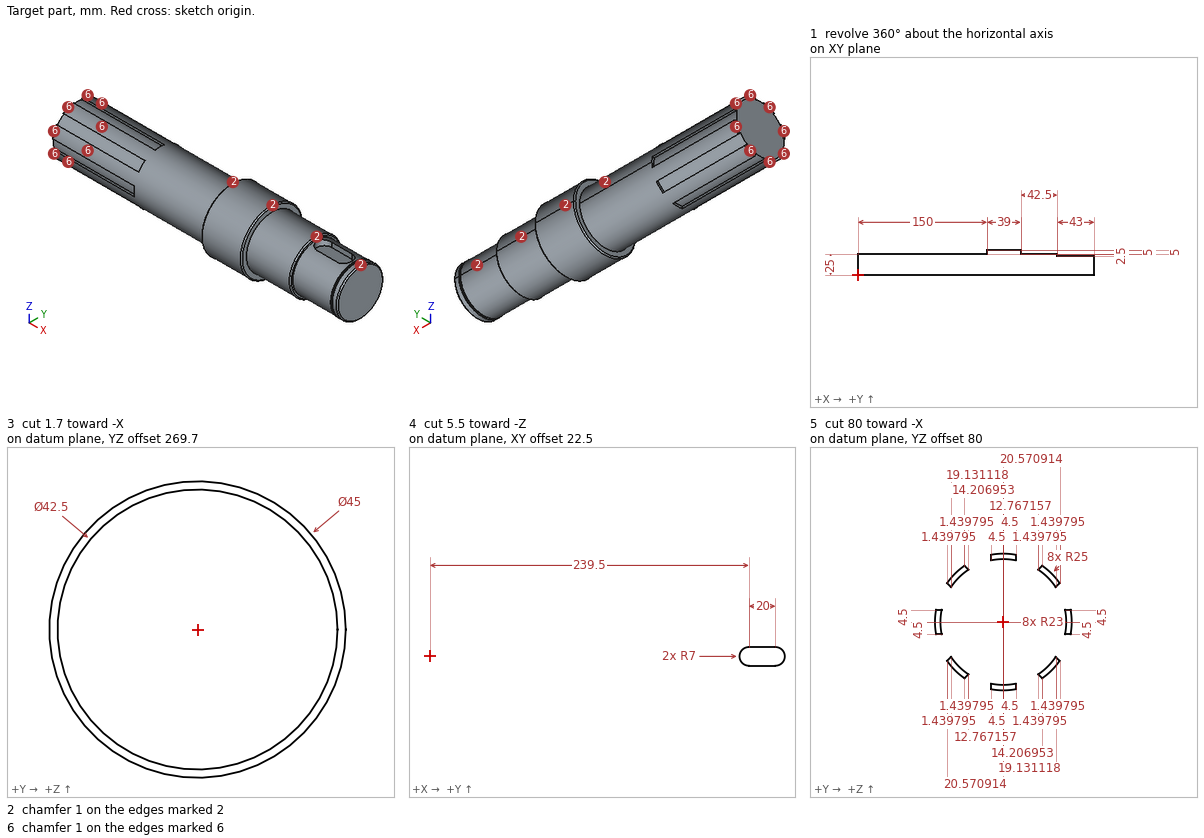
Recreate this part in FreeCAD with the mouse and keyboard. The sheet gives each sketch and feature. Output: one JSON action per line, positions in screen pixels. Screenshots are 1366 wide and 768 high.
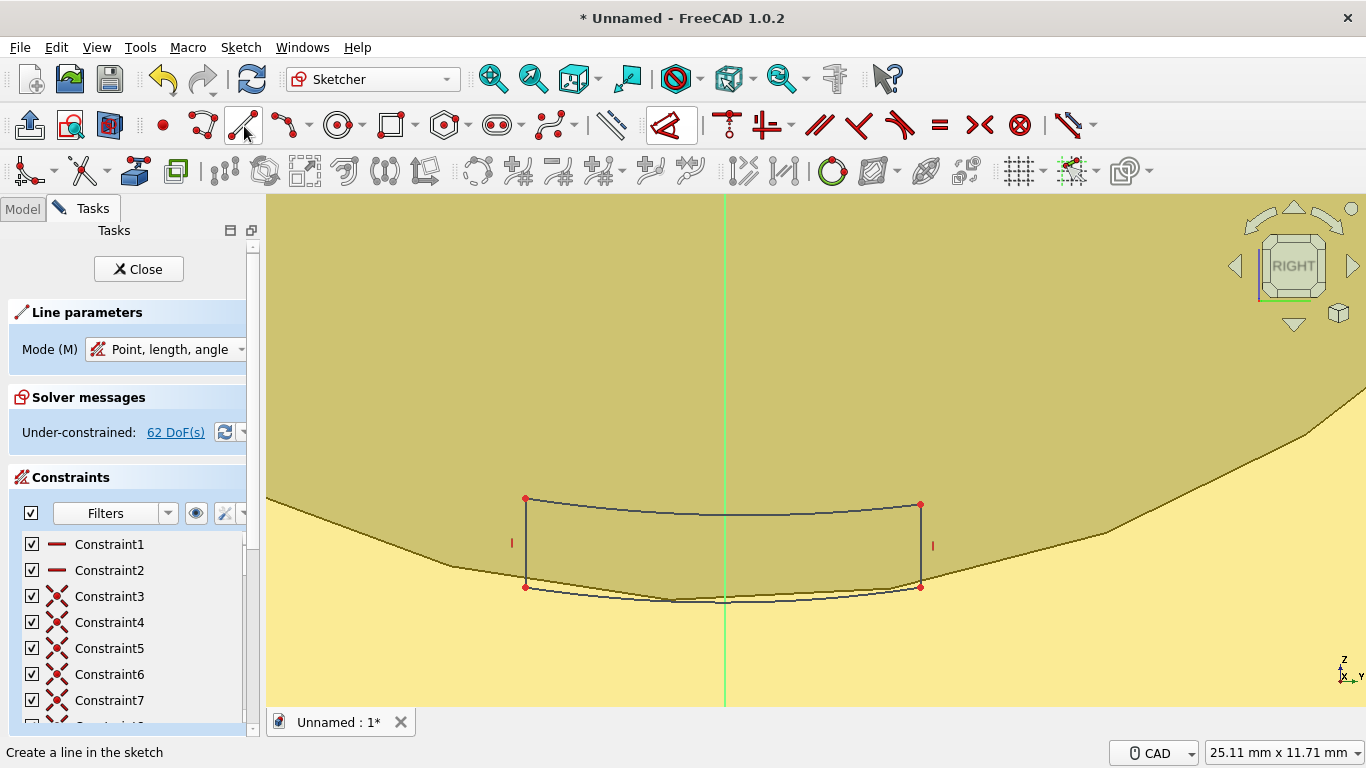
{"action": "scroll", "coordinate": [751, 598], "scroll_direction": "down", "scroll_amount": 10}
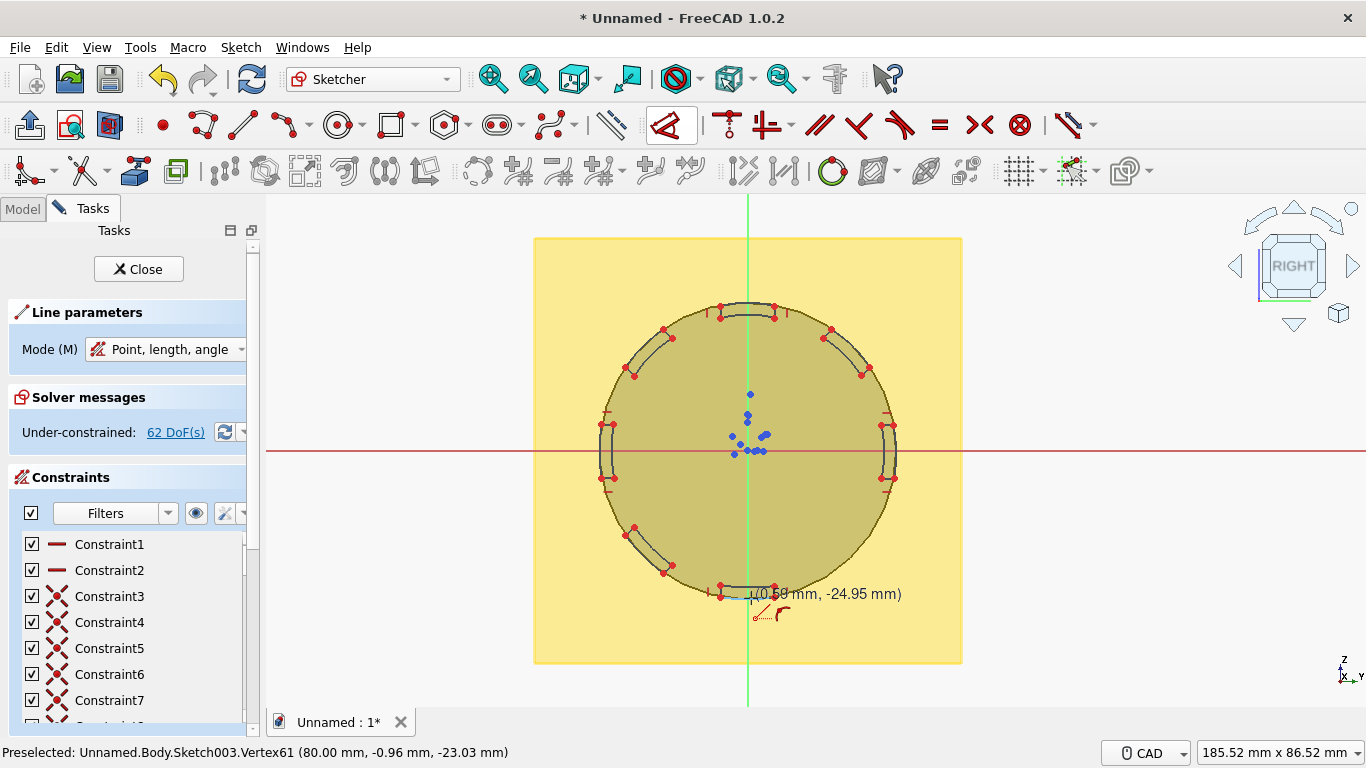
{"action": "left_click", "coordinate": [861, 527]}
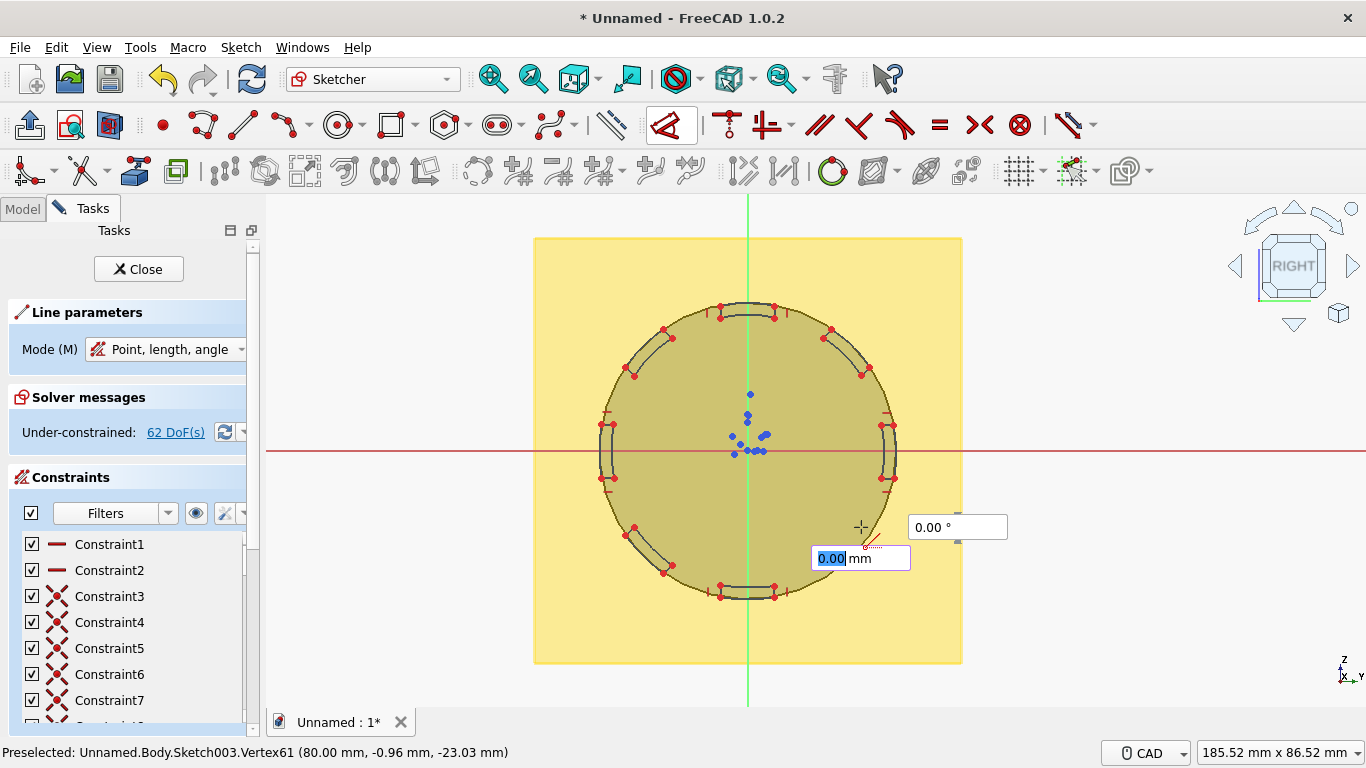
{"action": "scroll", "coordinate": [870, 535], "scroll_direction": "up", "scroll_amount": 2}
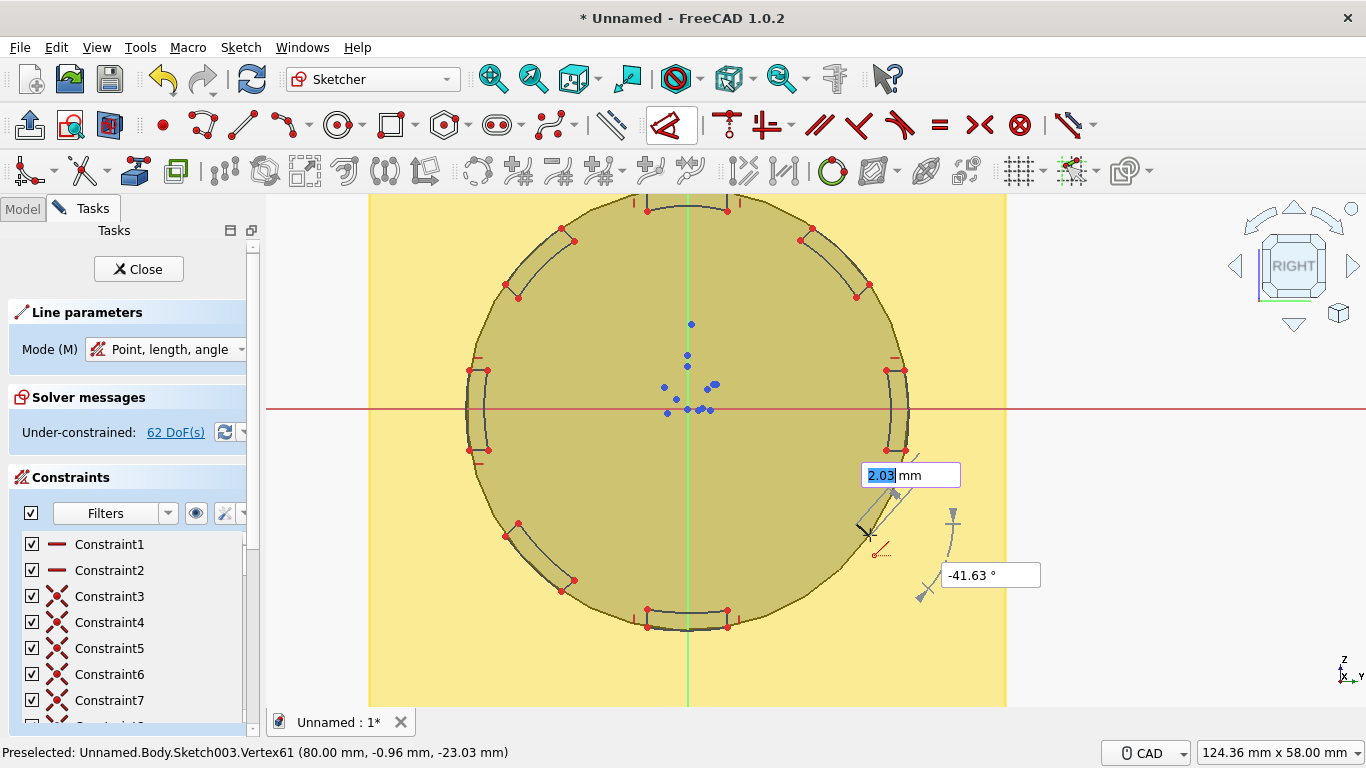
{"action": "left_click", "coordinate": [870, 535]}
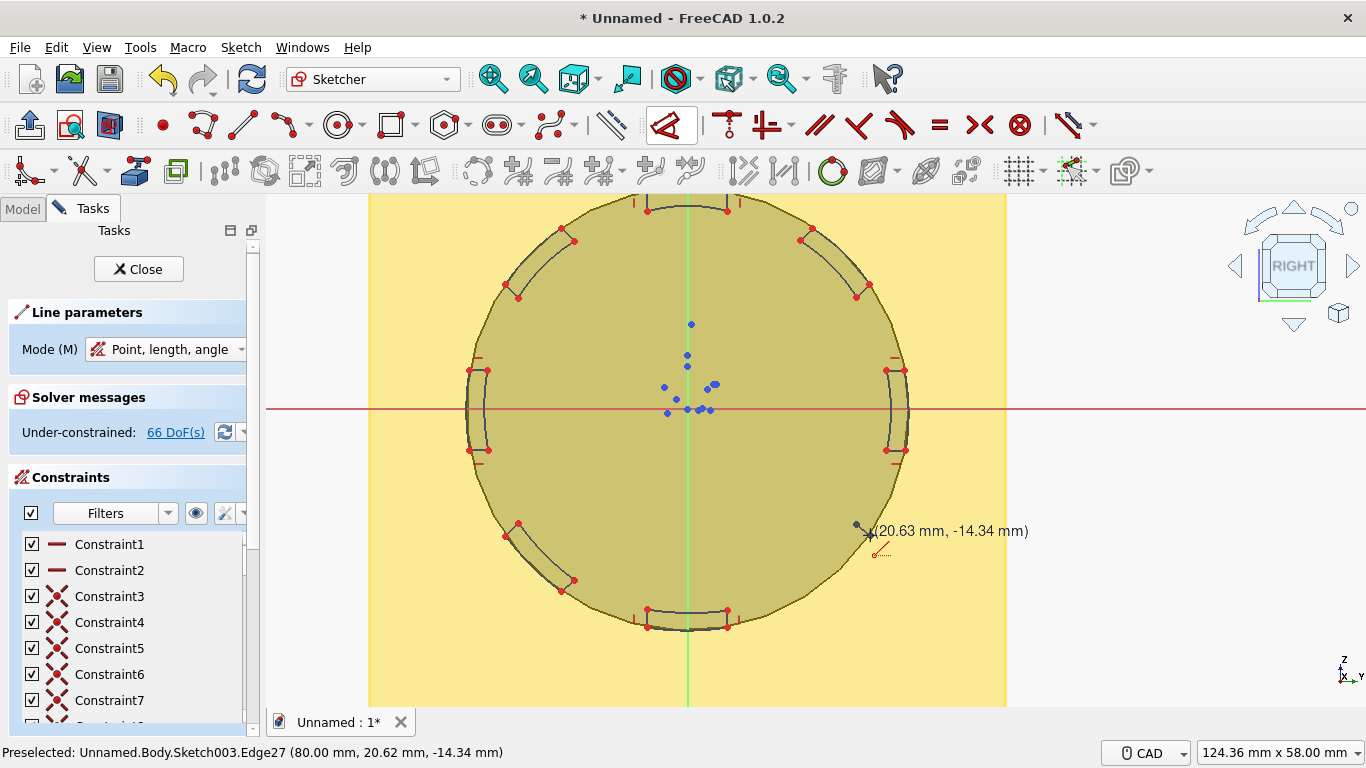
{"action": "left_click", "coordinate": [813, 591]}
{"action": "left_click", "coordinate": [800, 578]}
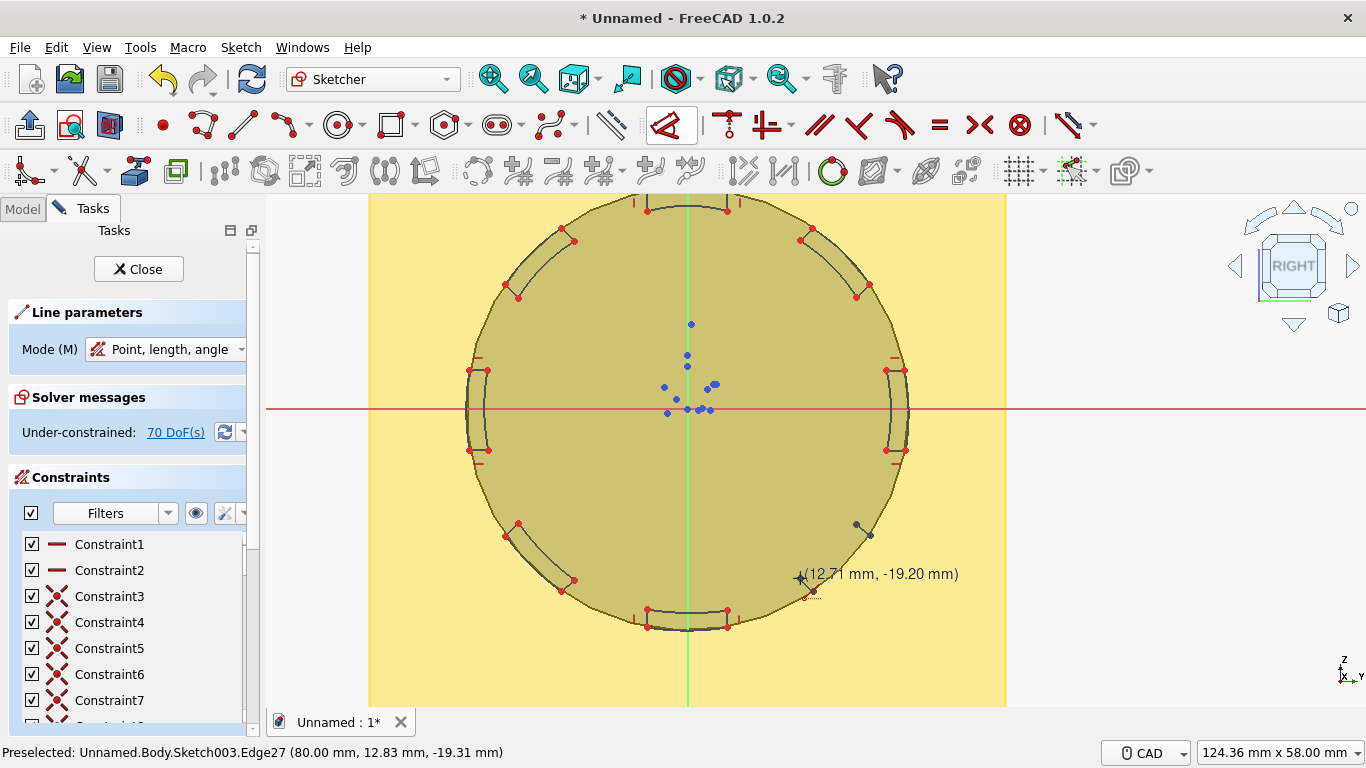
{"action": "left_click", "coordinate": [284, 126]}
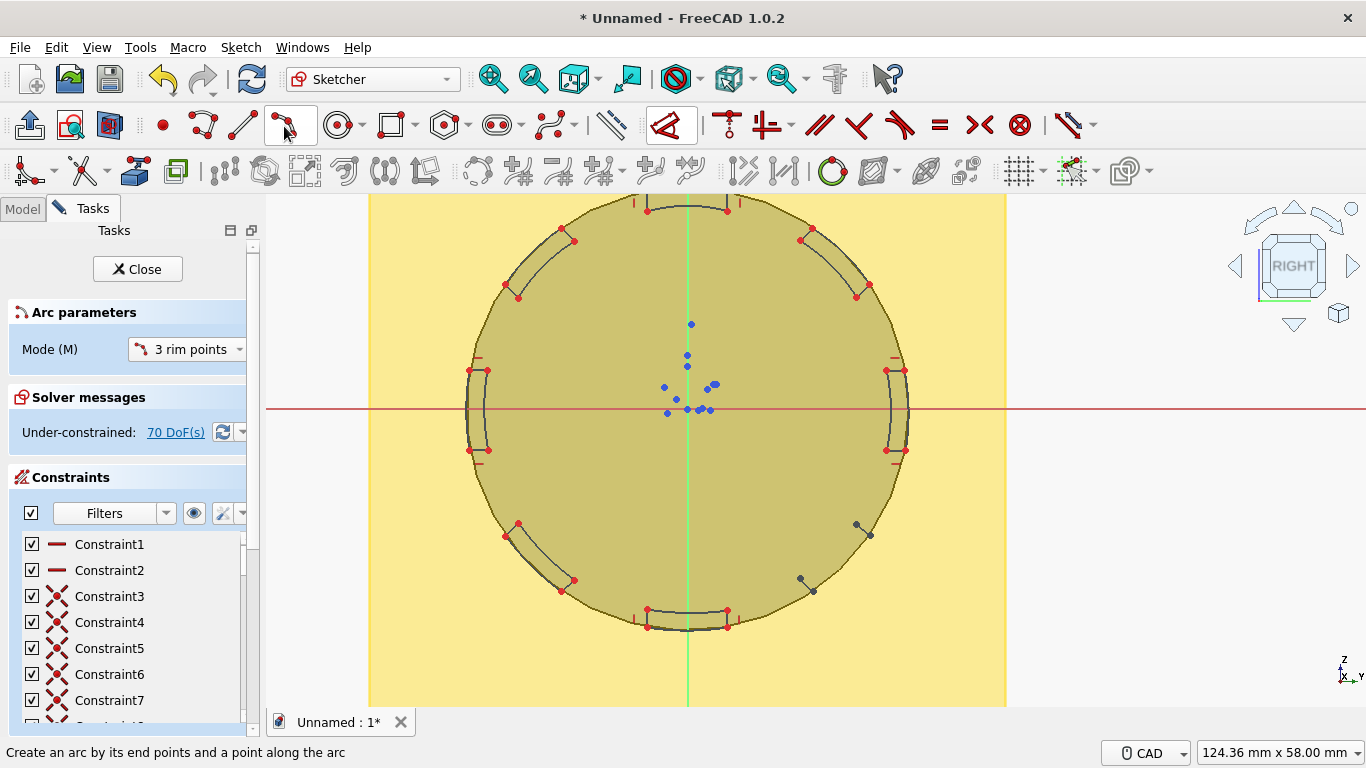
{"action": "scroll", "coordinate": [870, 535], "scroll_direction": "up", "scroll_amount": 3}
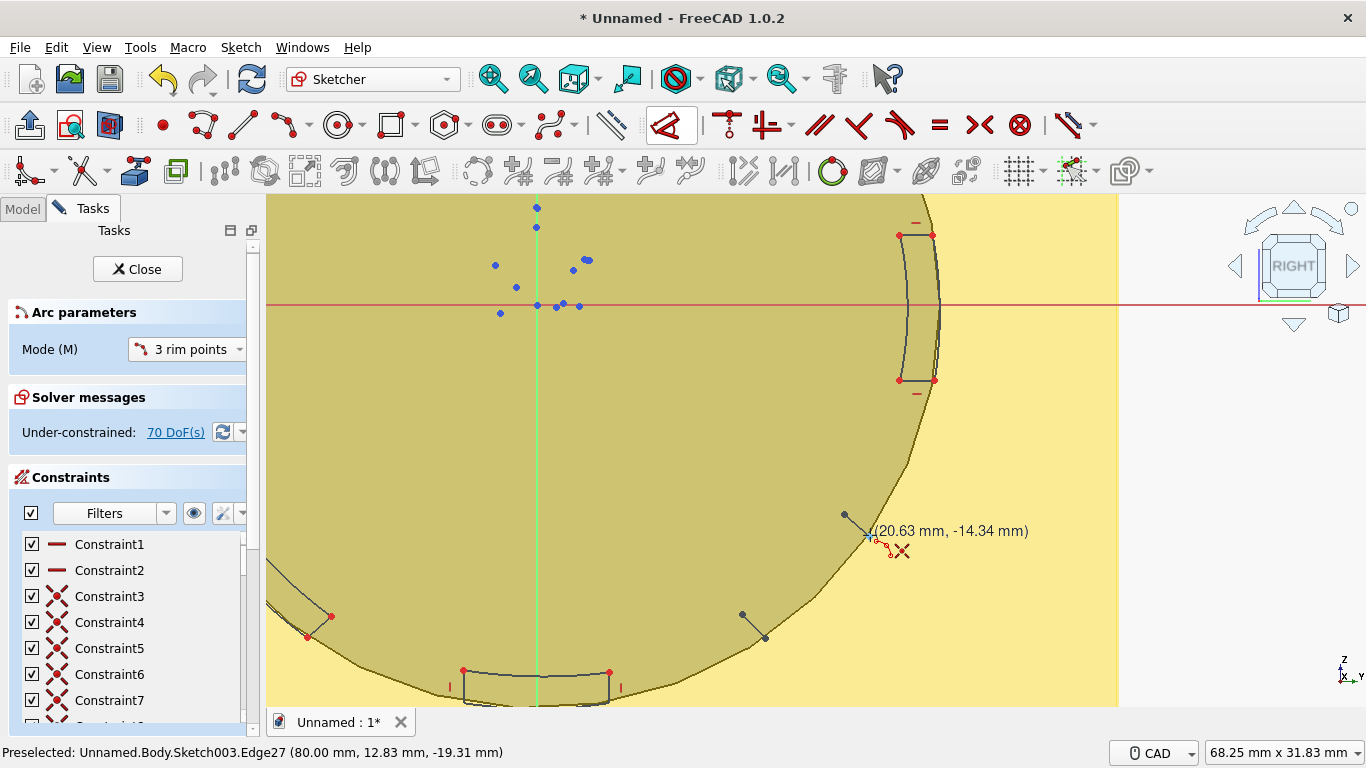
{"action": "left_click", "coordinate": [870, 536]}
{"action": "left_click", "coordinate": [766, 638]}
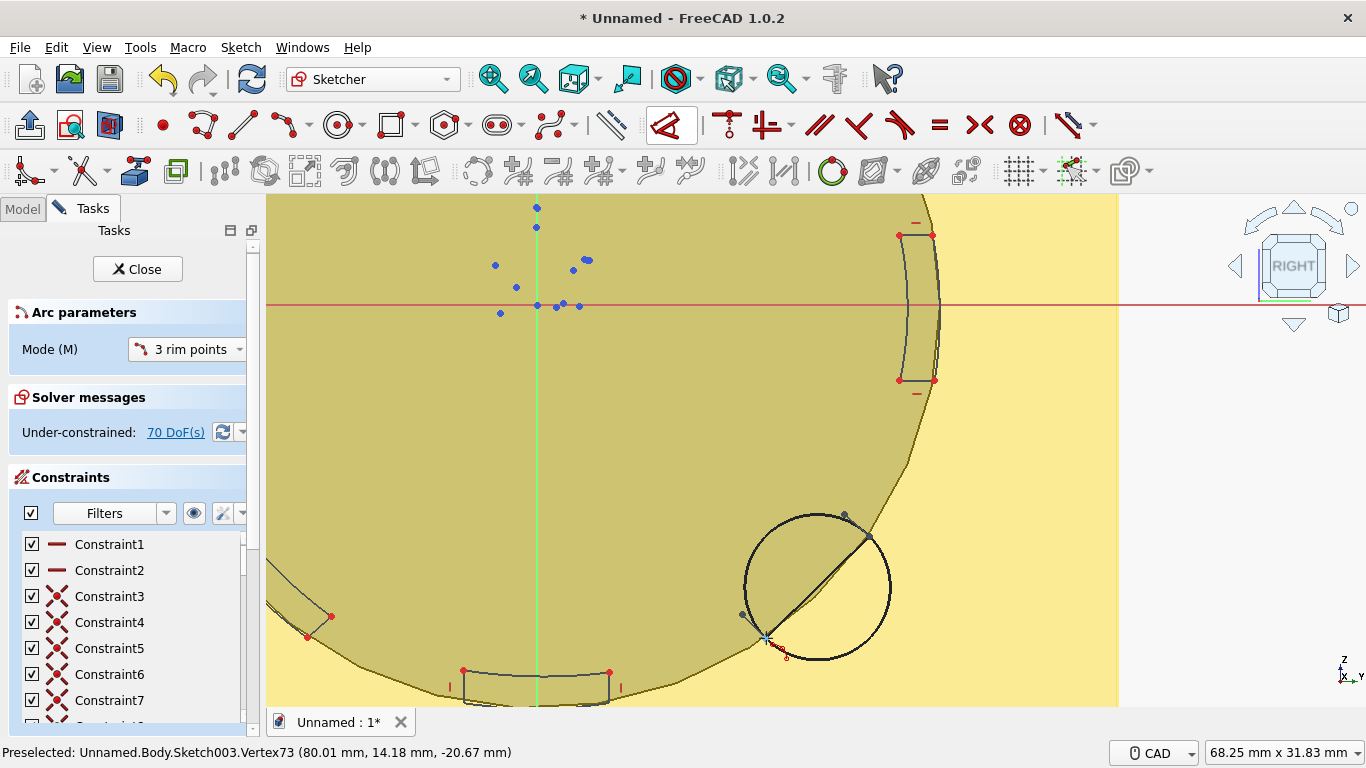
{"action": "scroll", "coordinate": [822, 590], "scroll_direction": "up", "scroll_amount": 5}